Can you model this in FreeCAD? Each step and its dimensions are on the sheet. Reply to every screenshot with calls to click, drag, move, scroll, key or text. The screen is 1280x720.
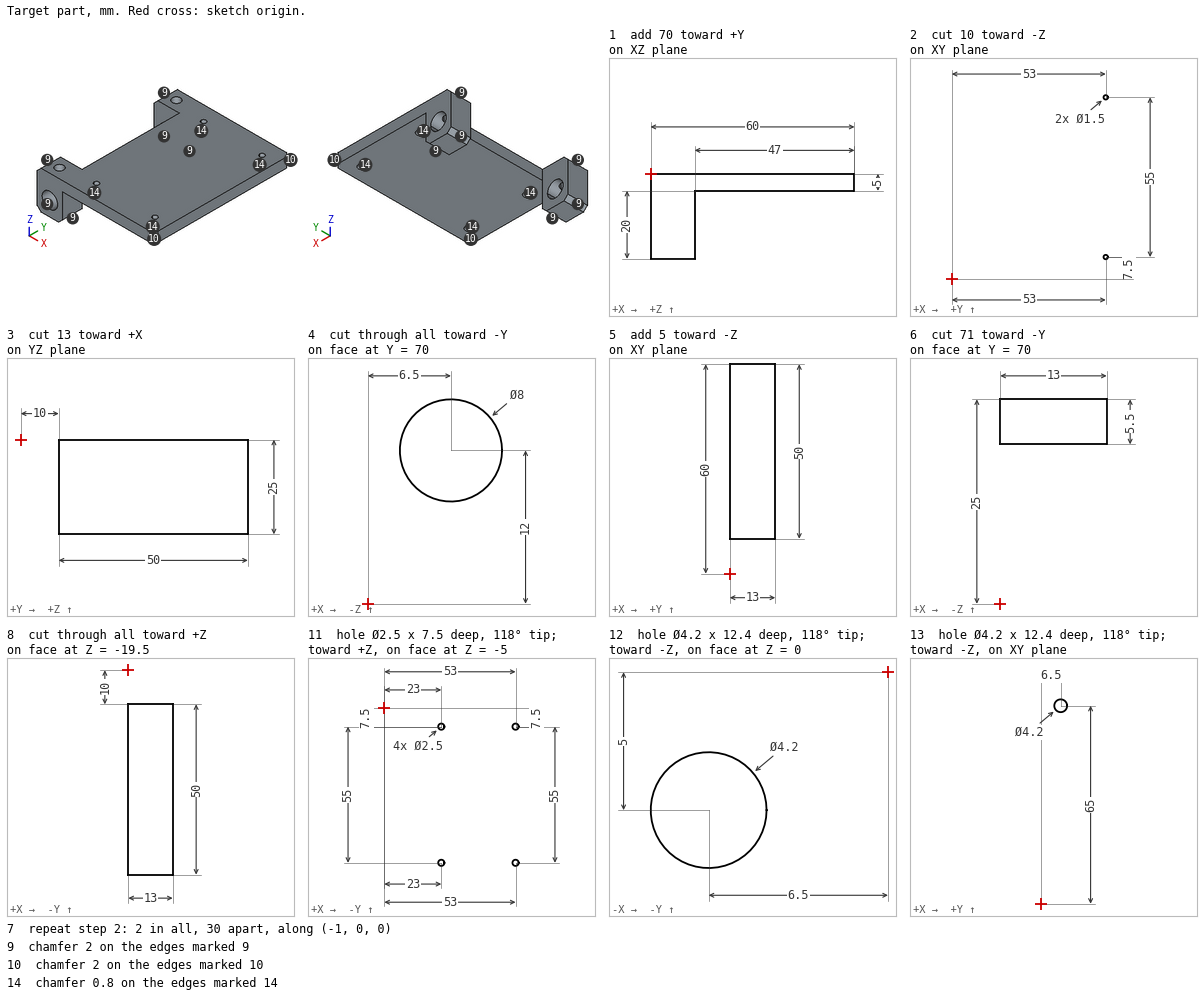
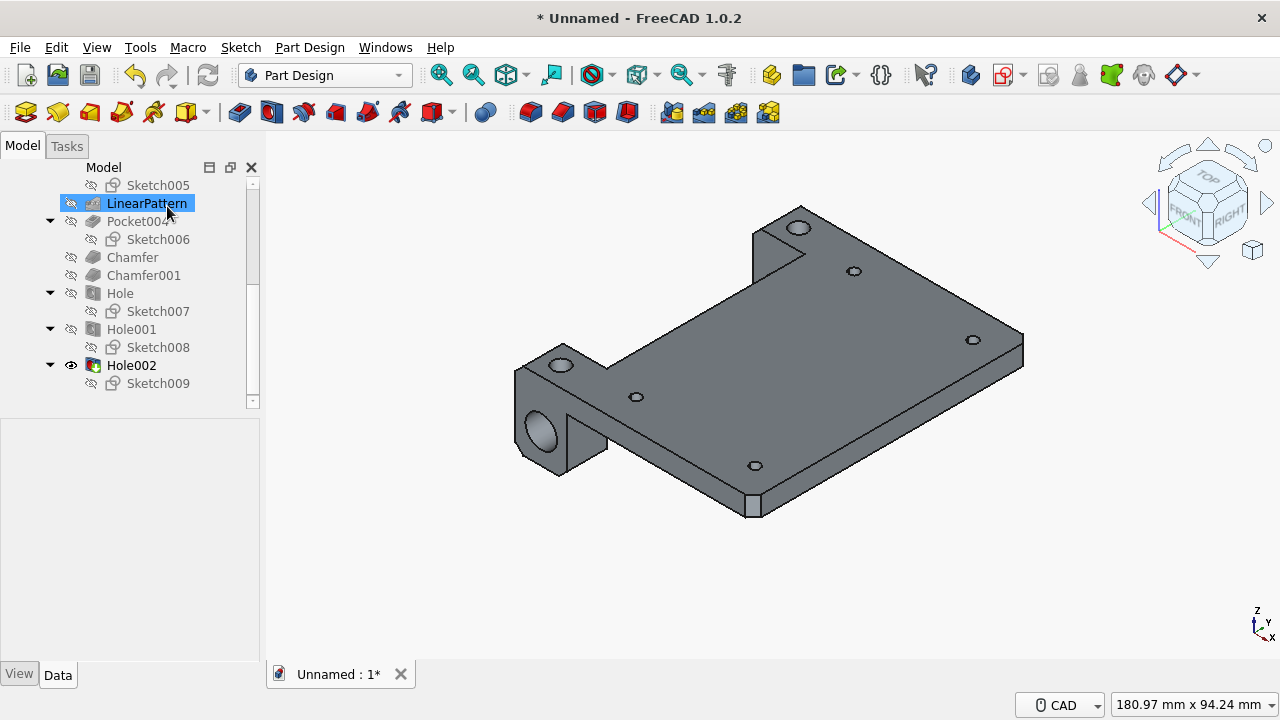
key(1)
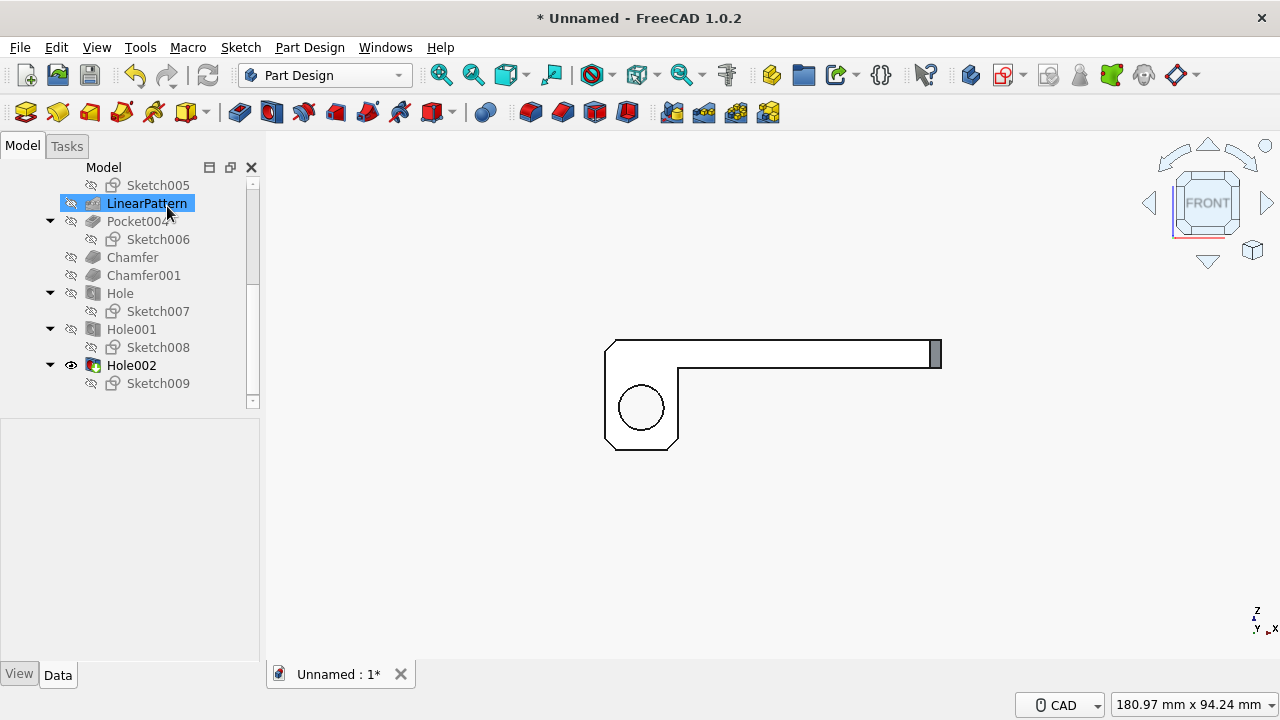
key(v)
key(f)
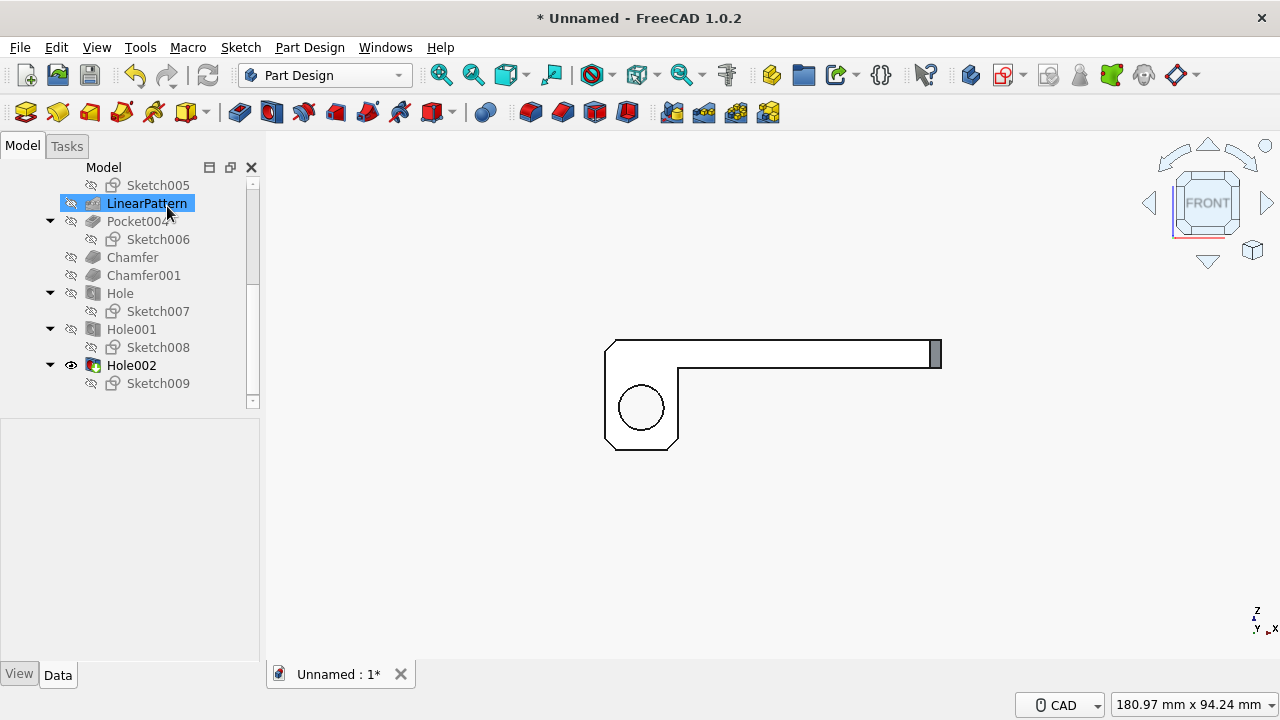
key(3)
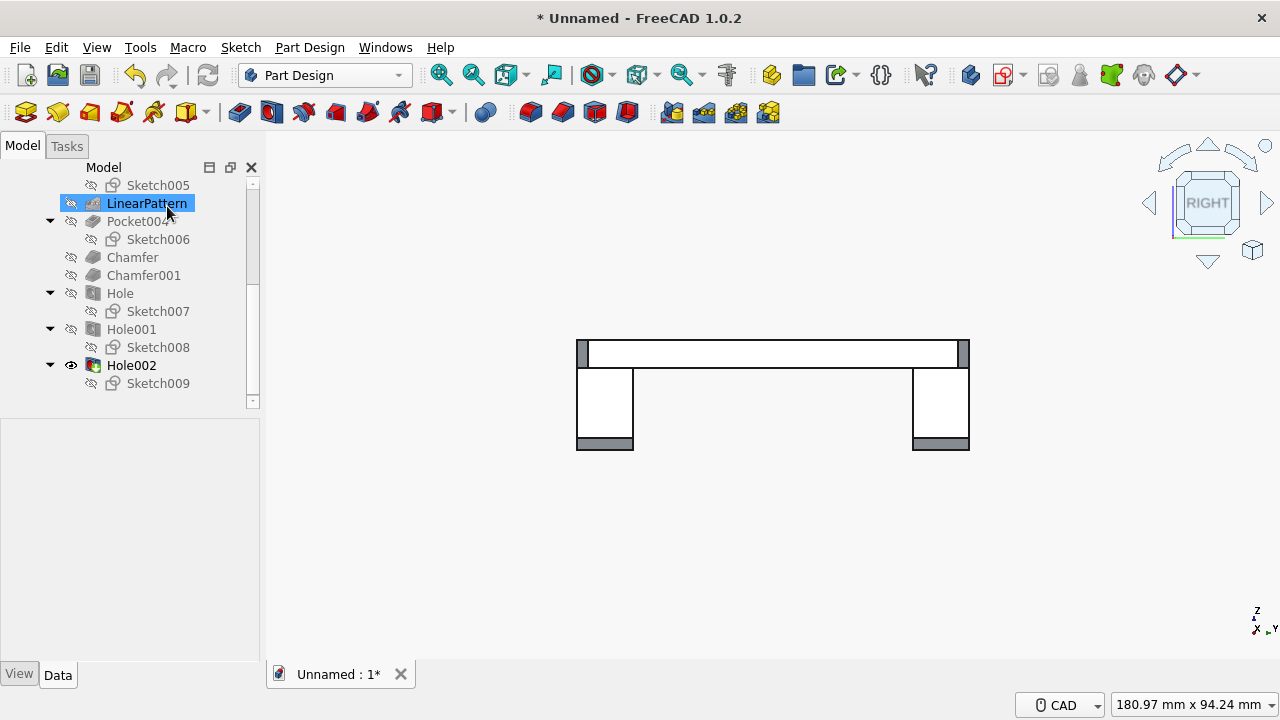
key(v)
key(f)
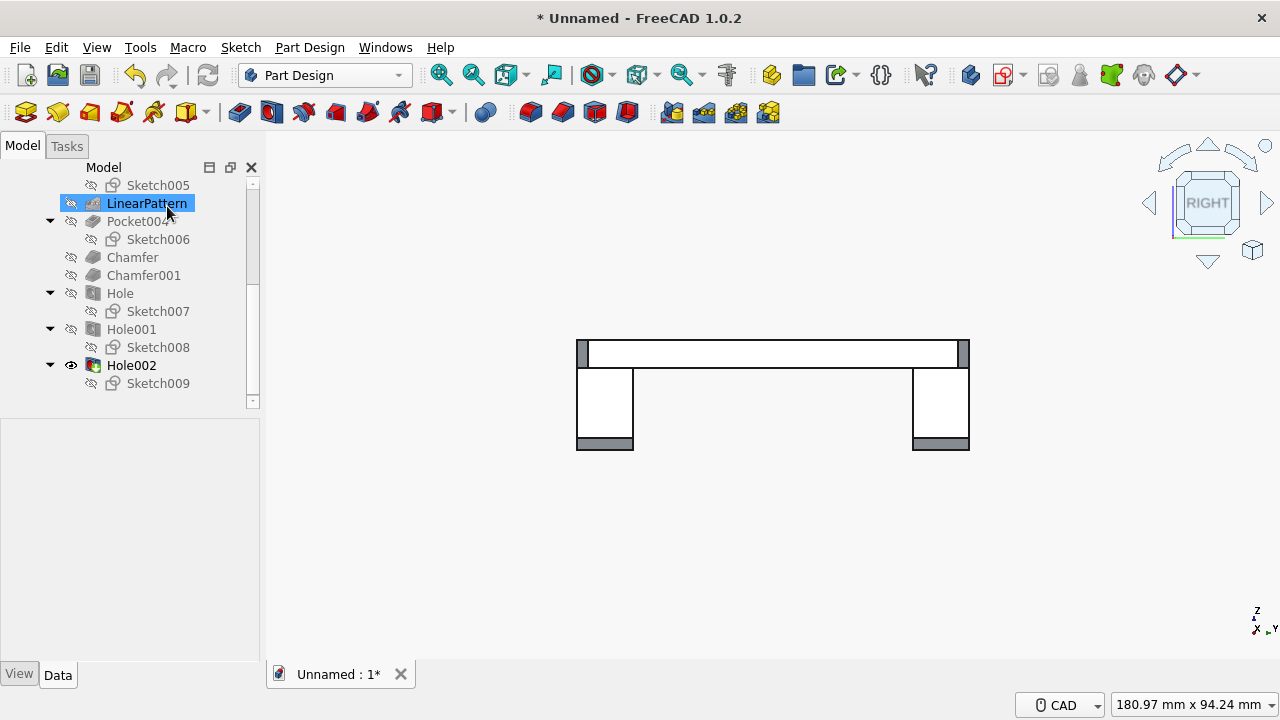
key(5)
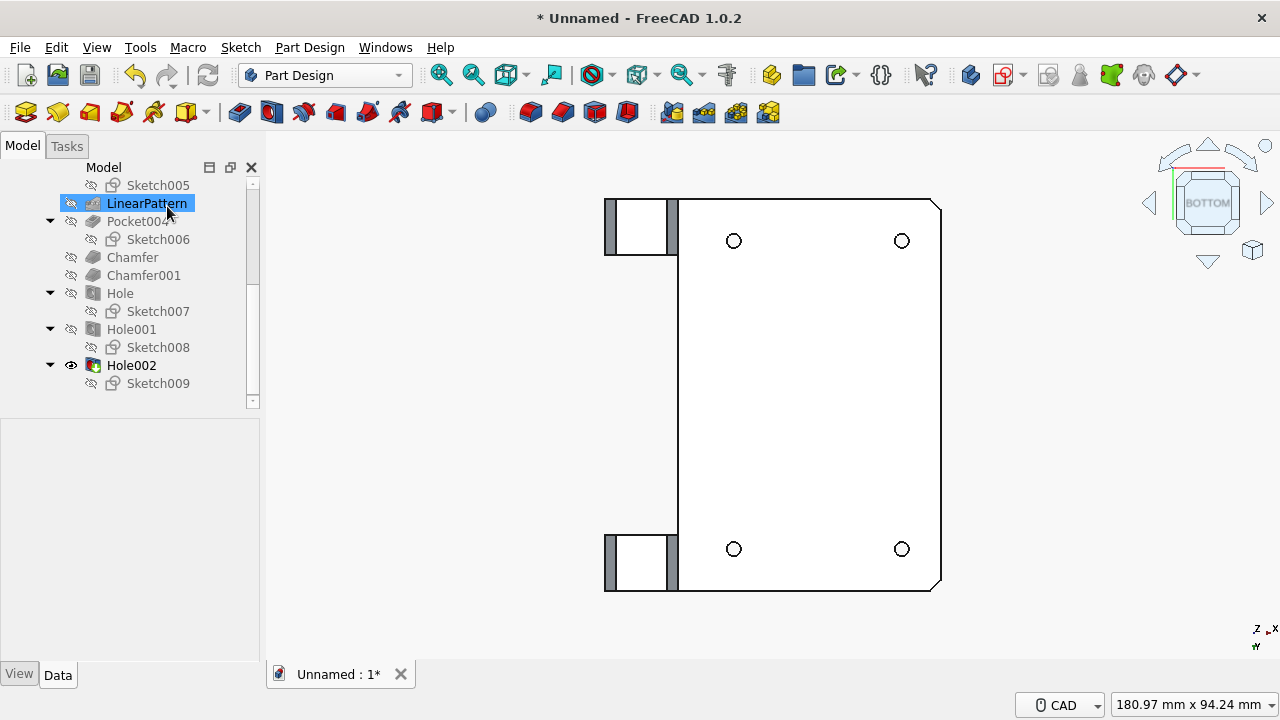
click(741, 548)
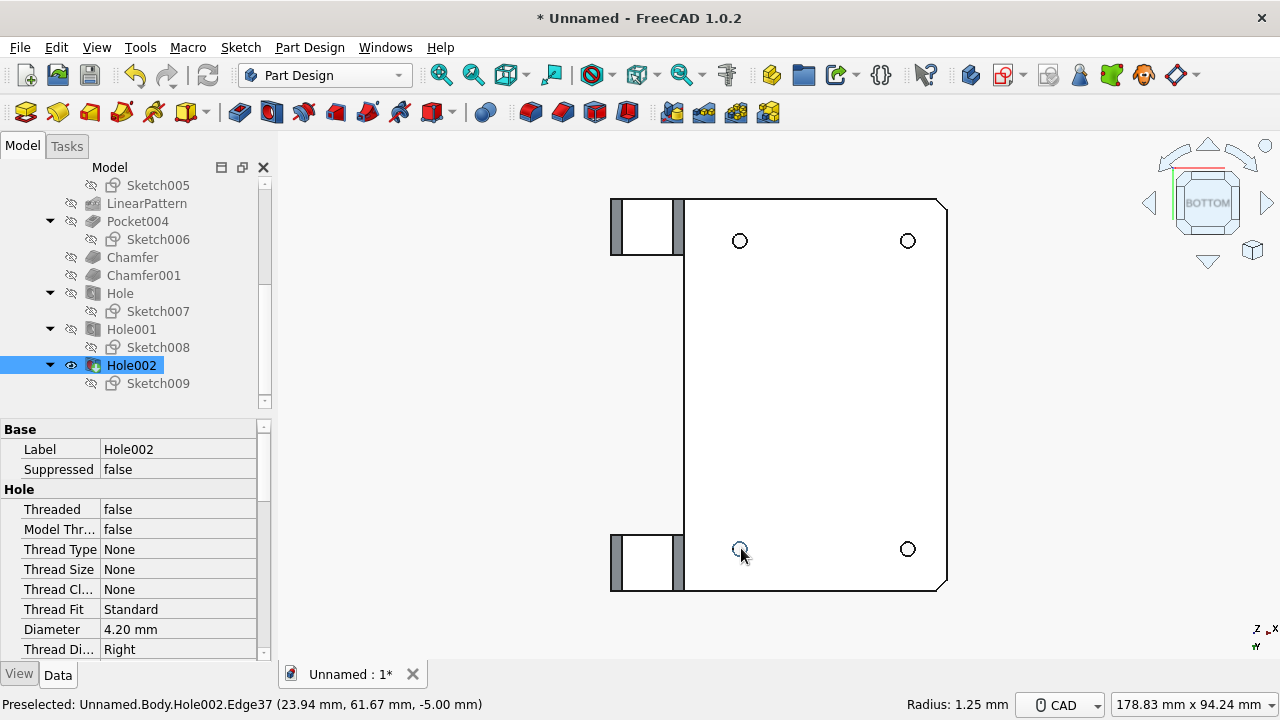
click(915, 548, ctrl)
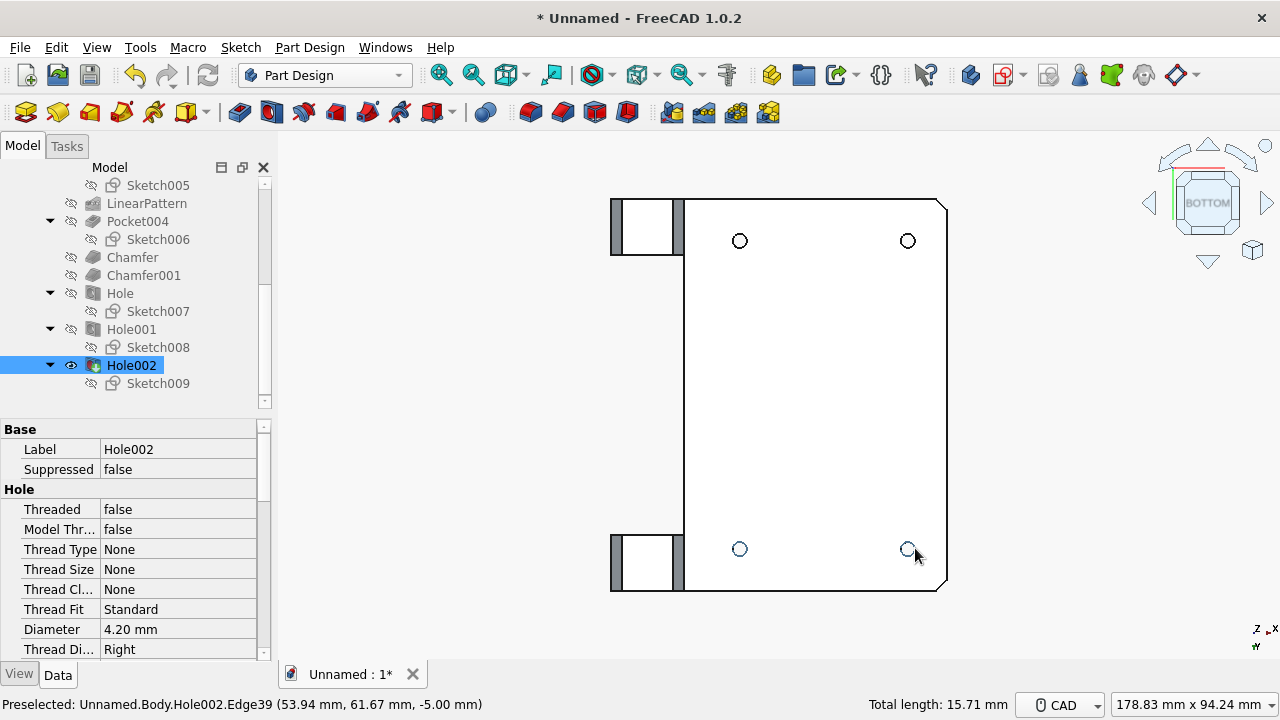
click(915, 240, ctrl)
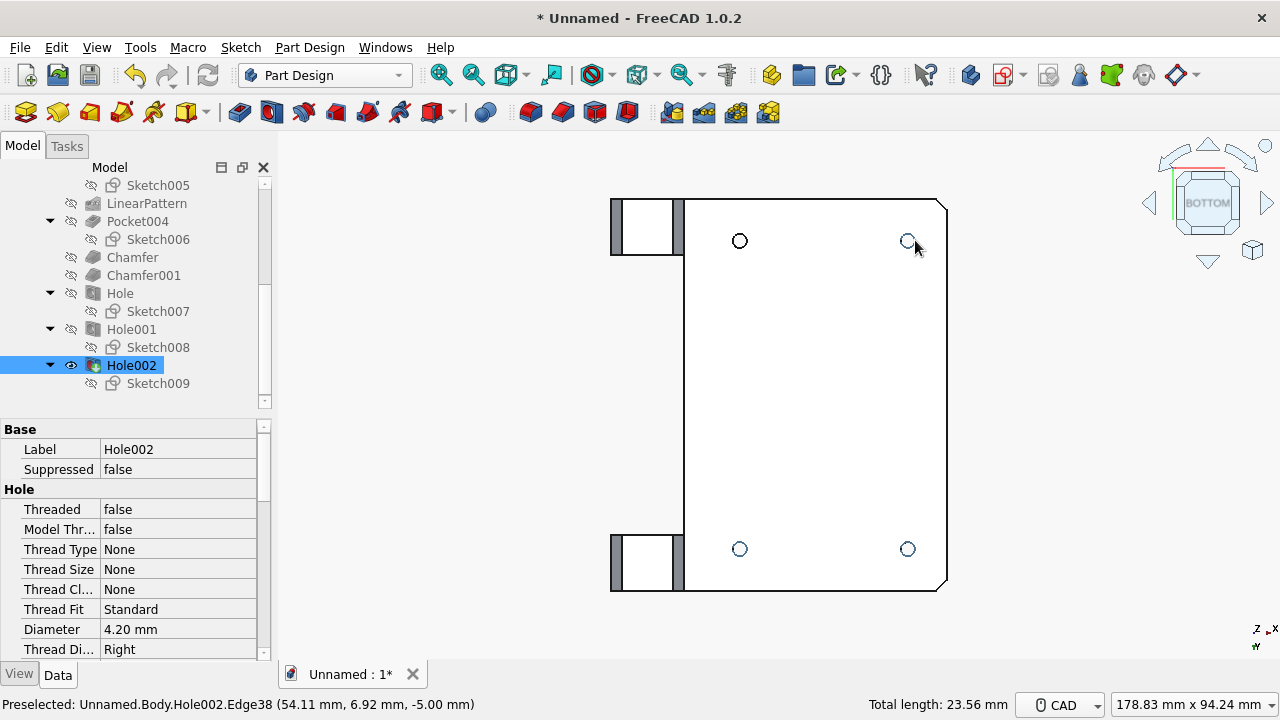
click(747, 240, ctrl)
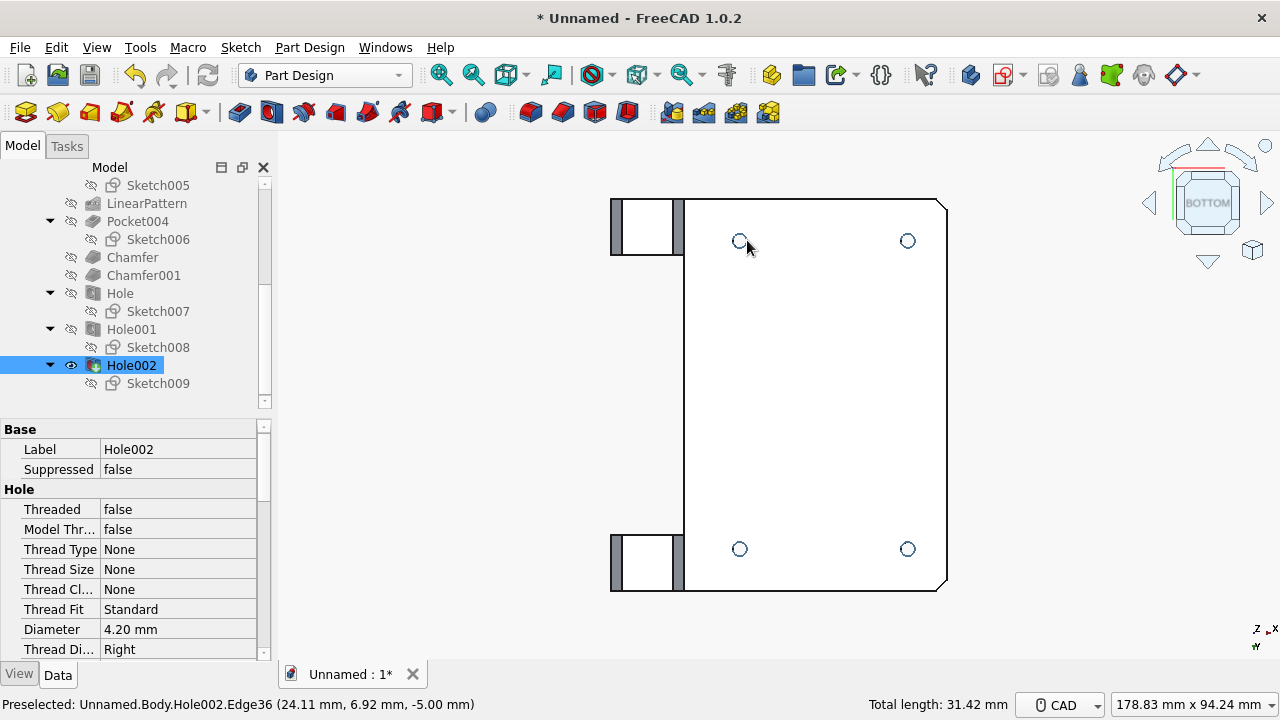
click(564, 112)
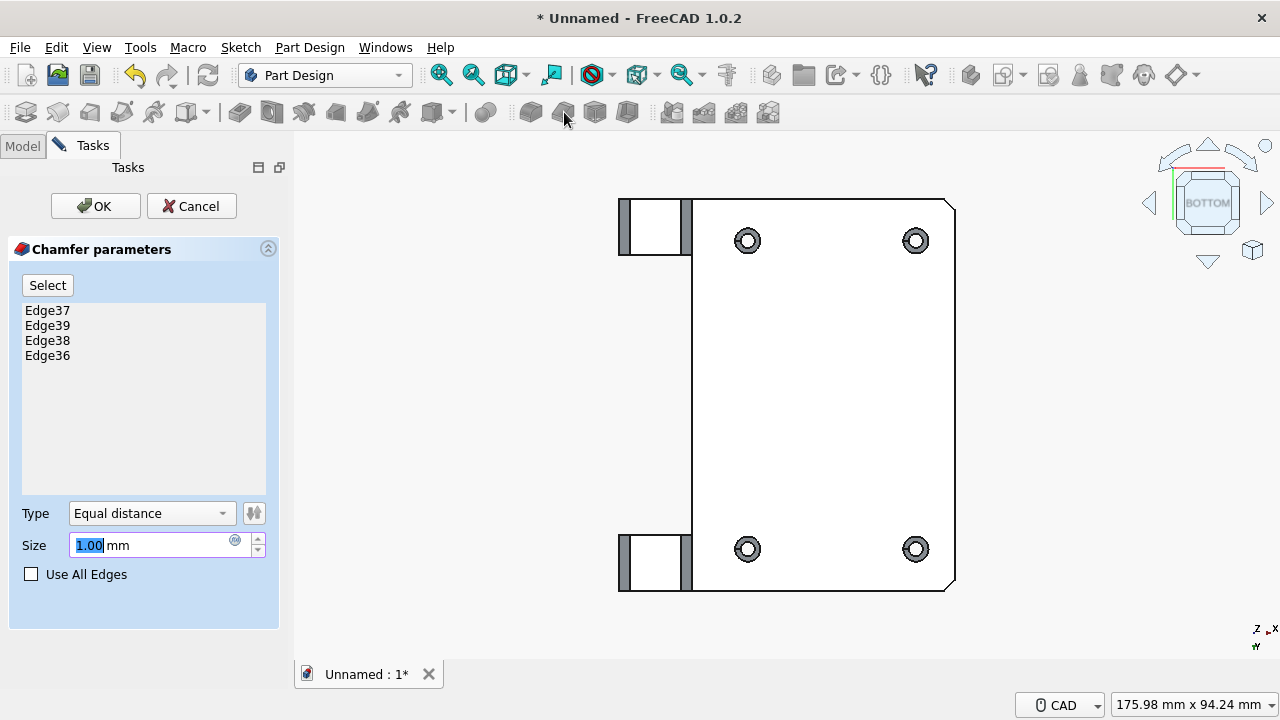
text(0.8)
key(Tab)